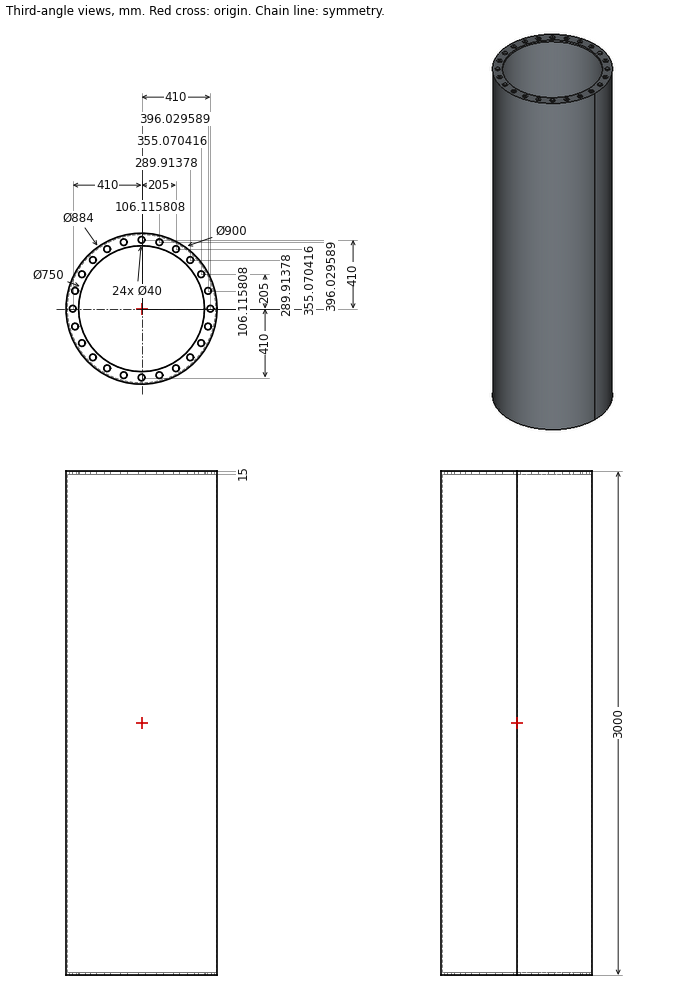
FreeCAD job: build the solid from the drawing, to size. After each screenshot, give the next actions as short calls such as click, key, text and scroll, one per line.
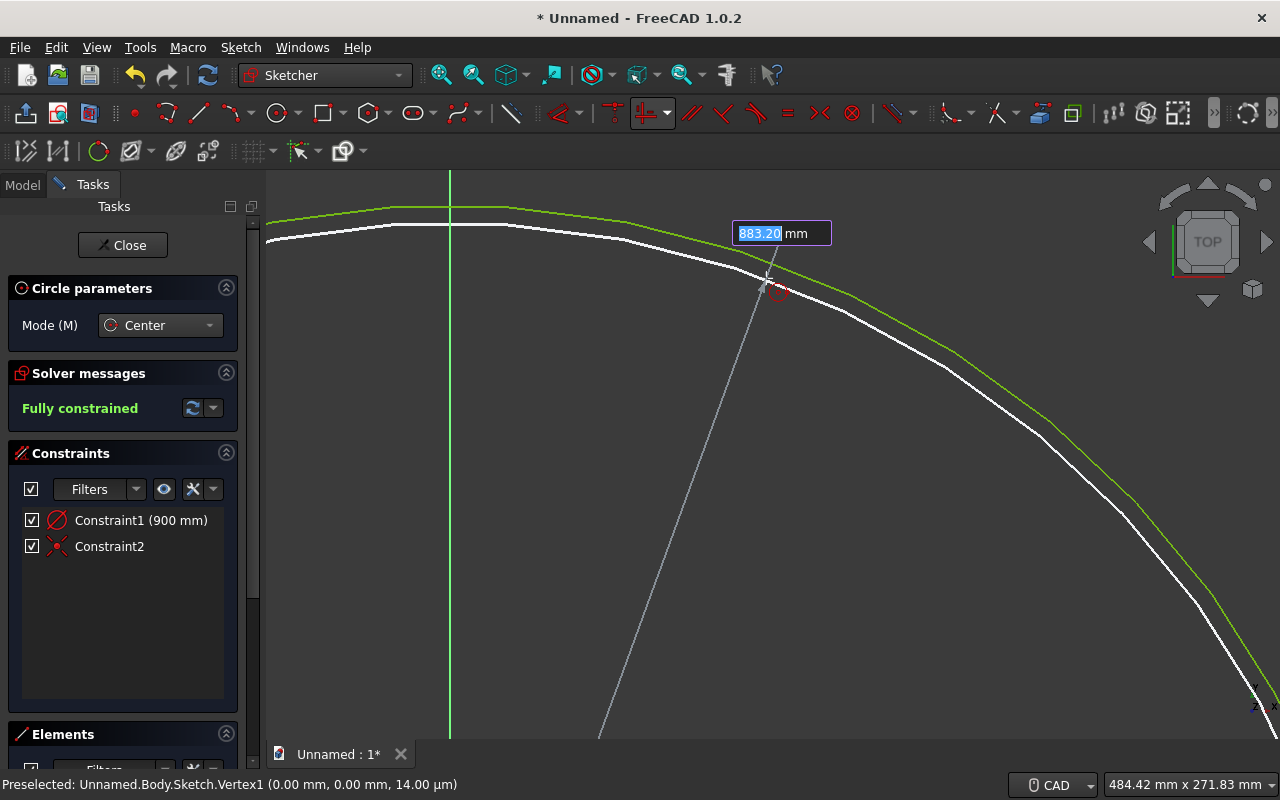
text(884)
key(Return)
key(Escape)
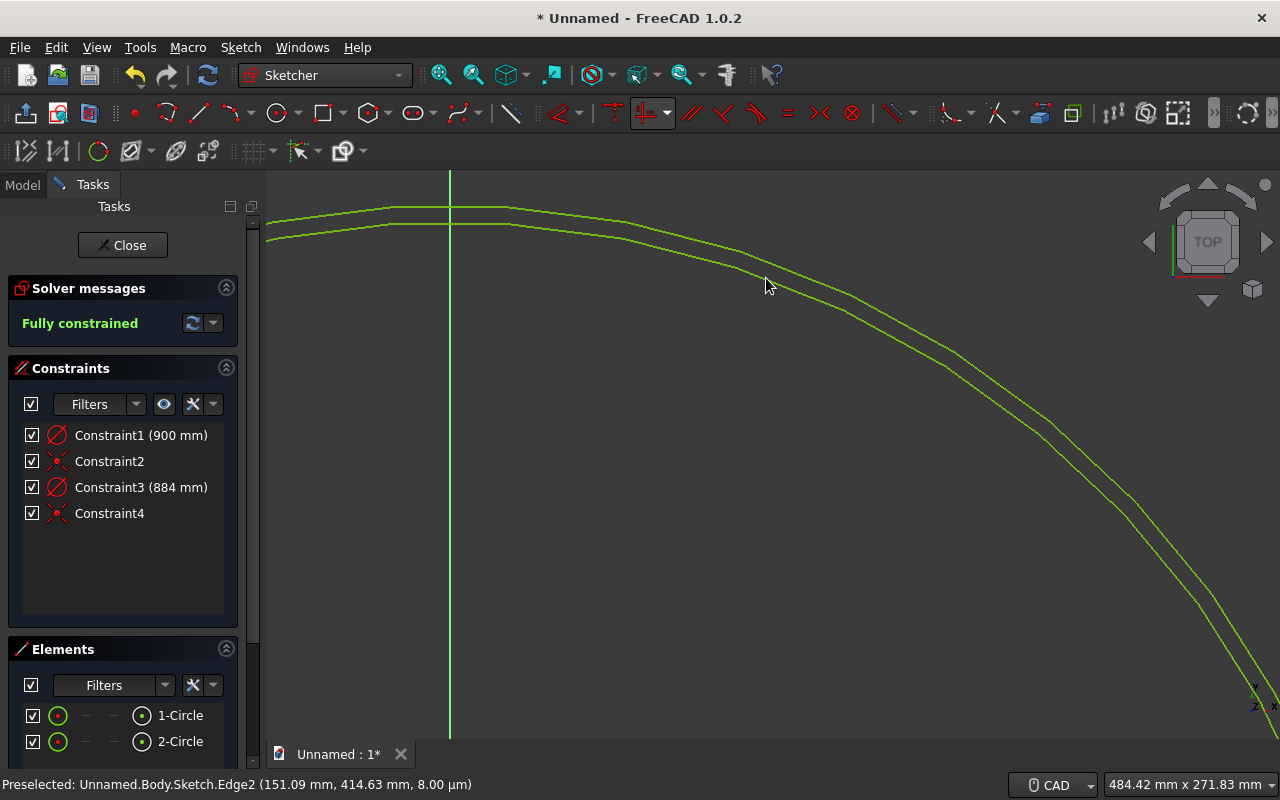
click(123, 245)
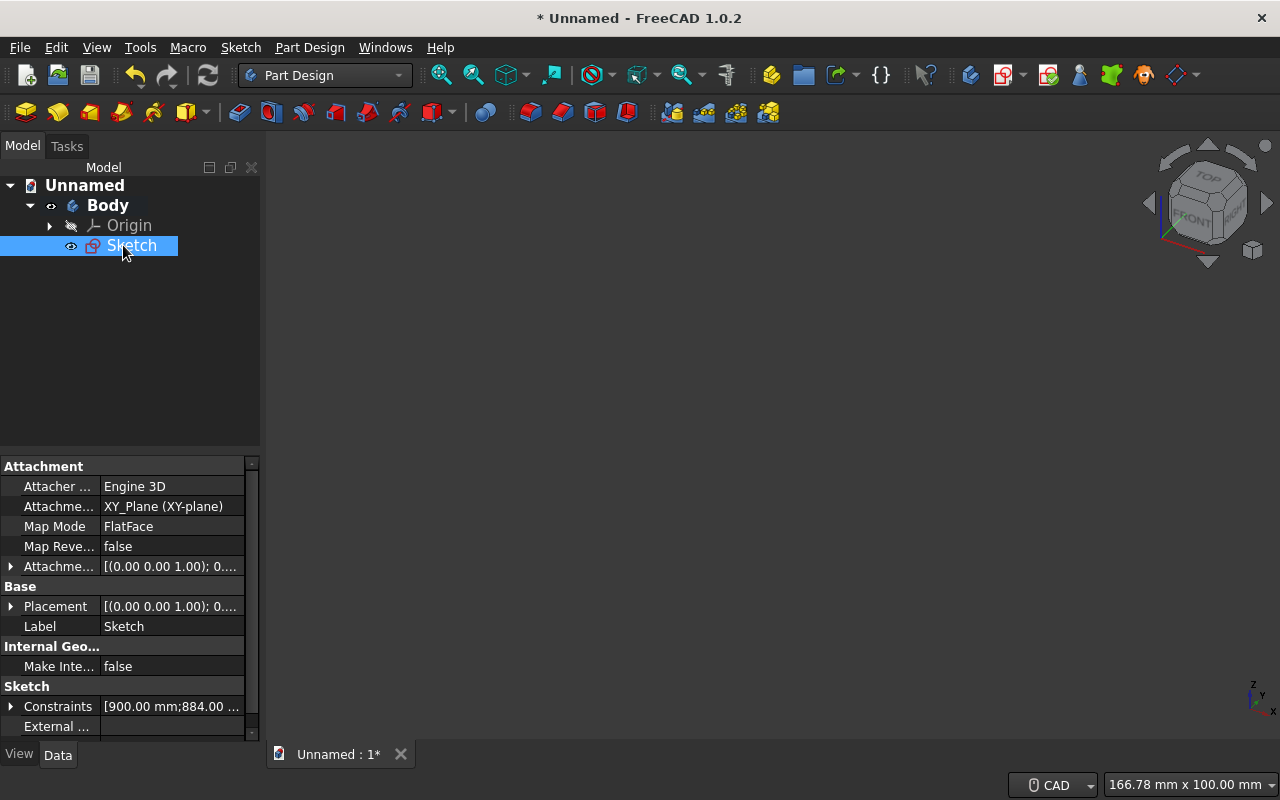
click(26, 112)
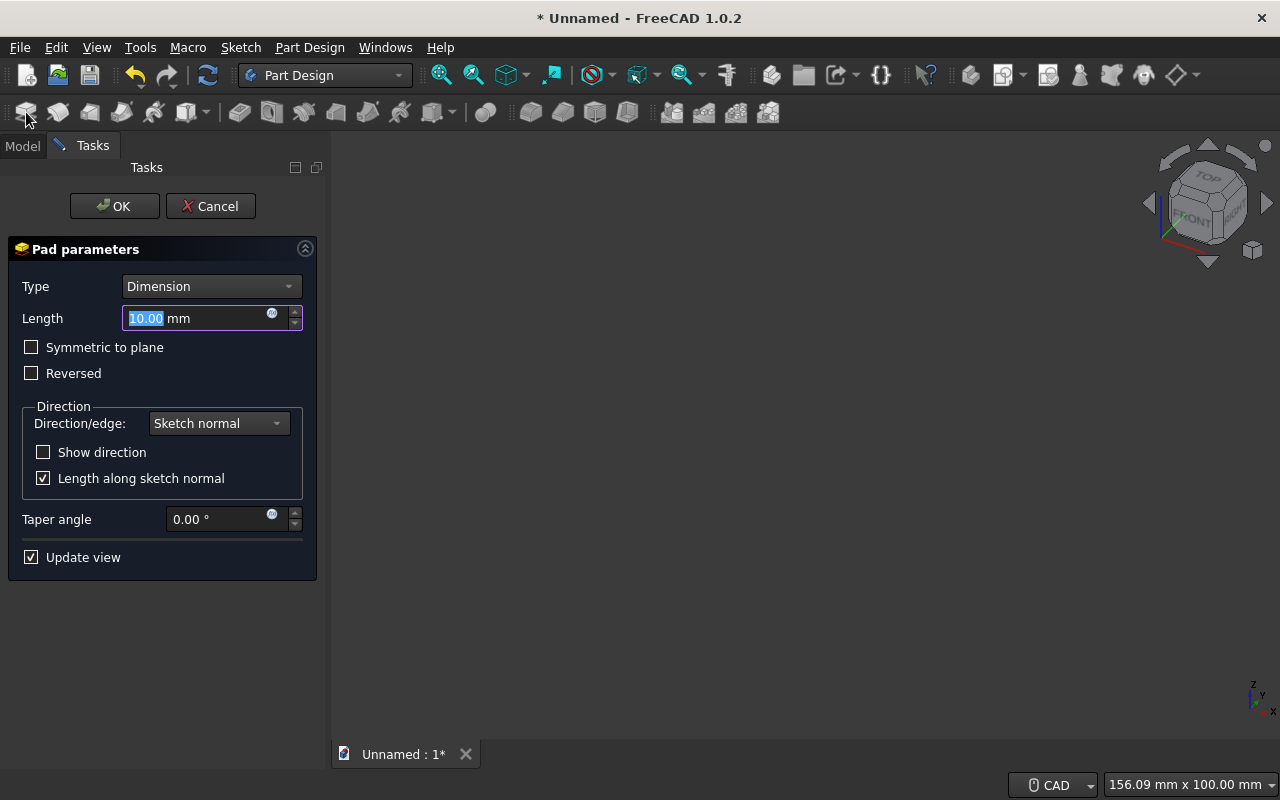
text(3000)
key(Tab)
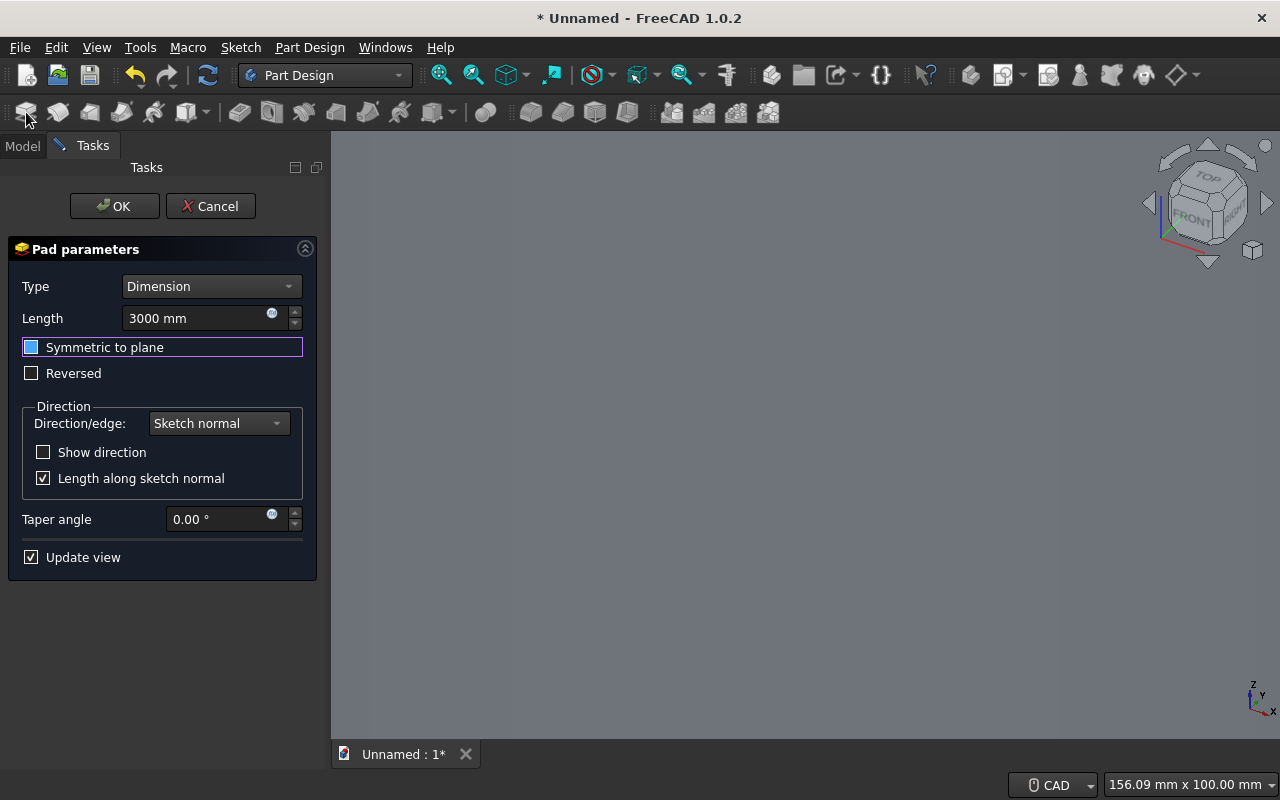
click(30, 347)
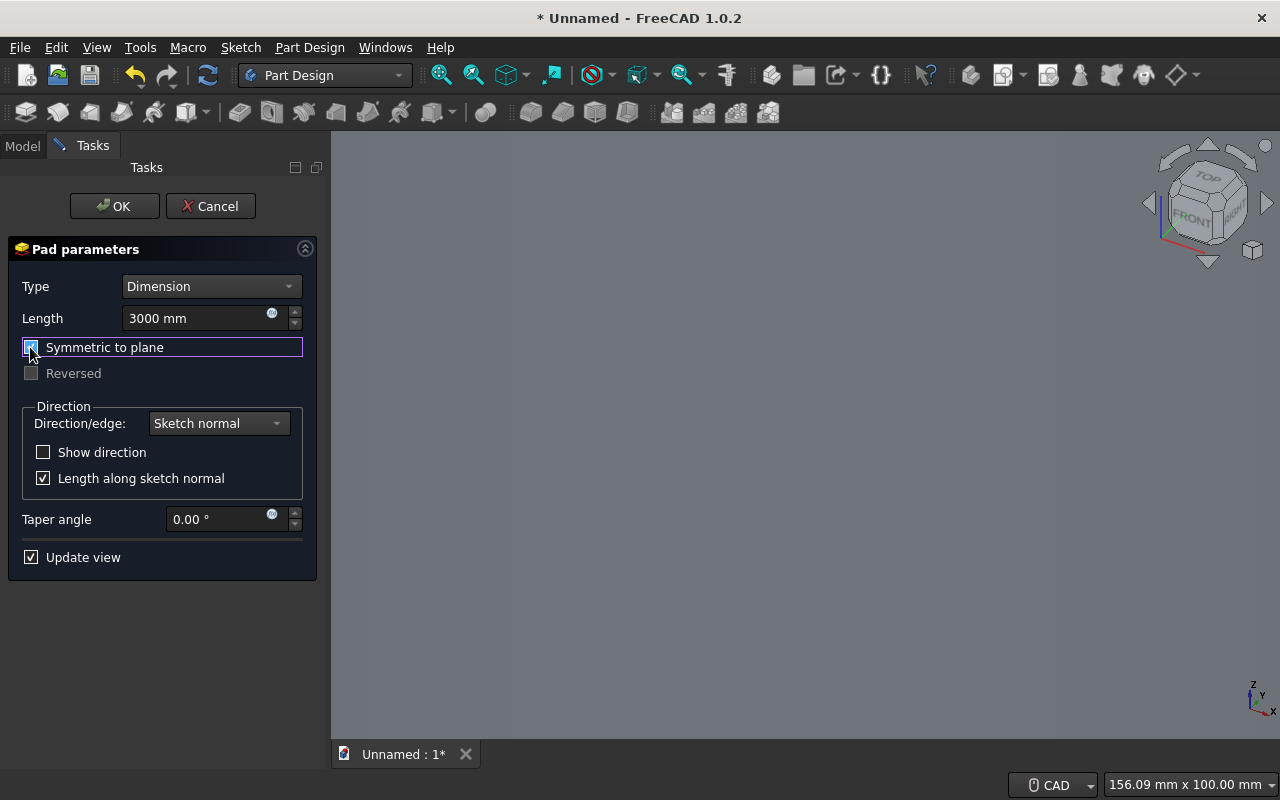
click(115, 206)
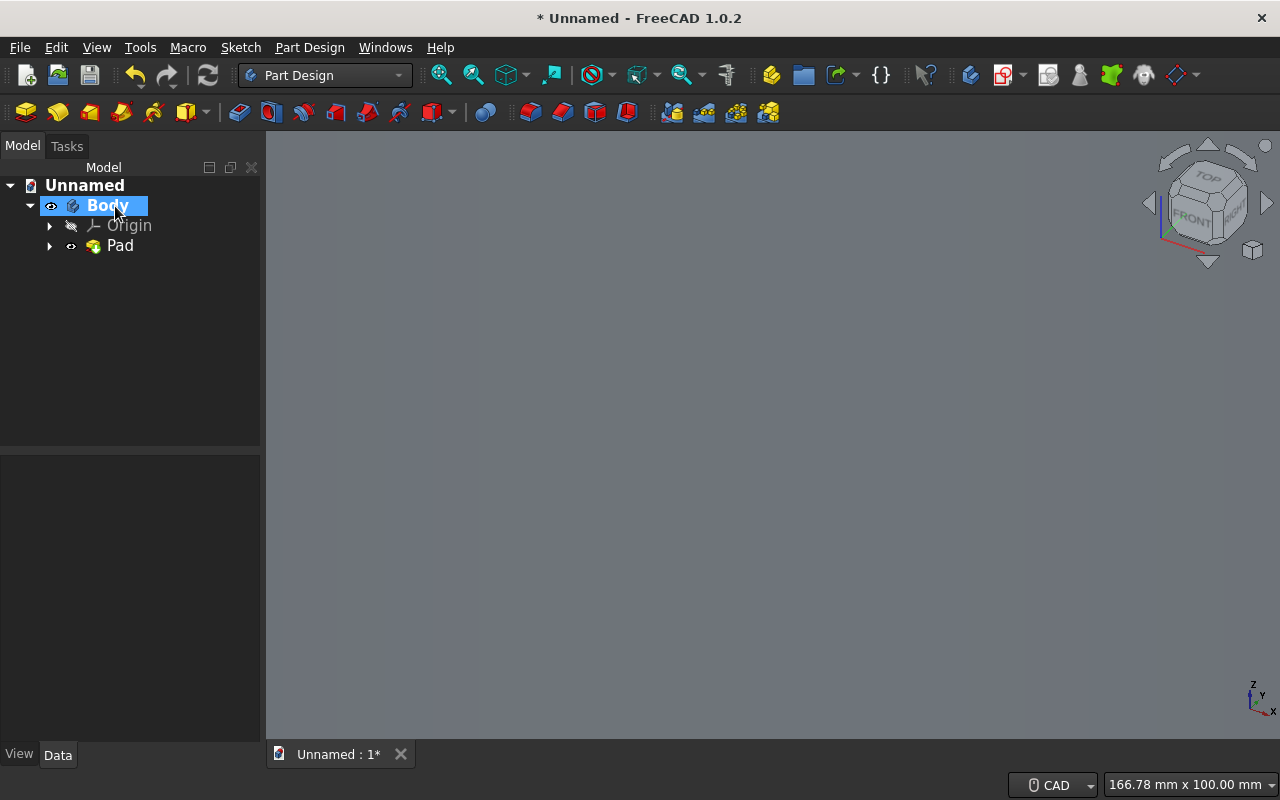
click(442, 76)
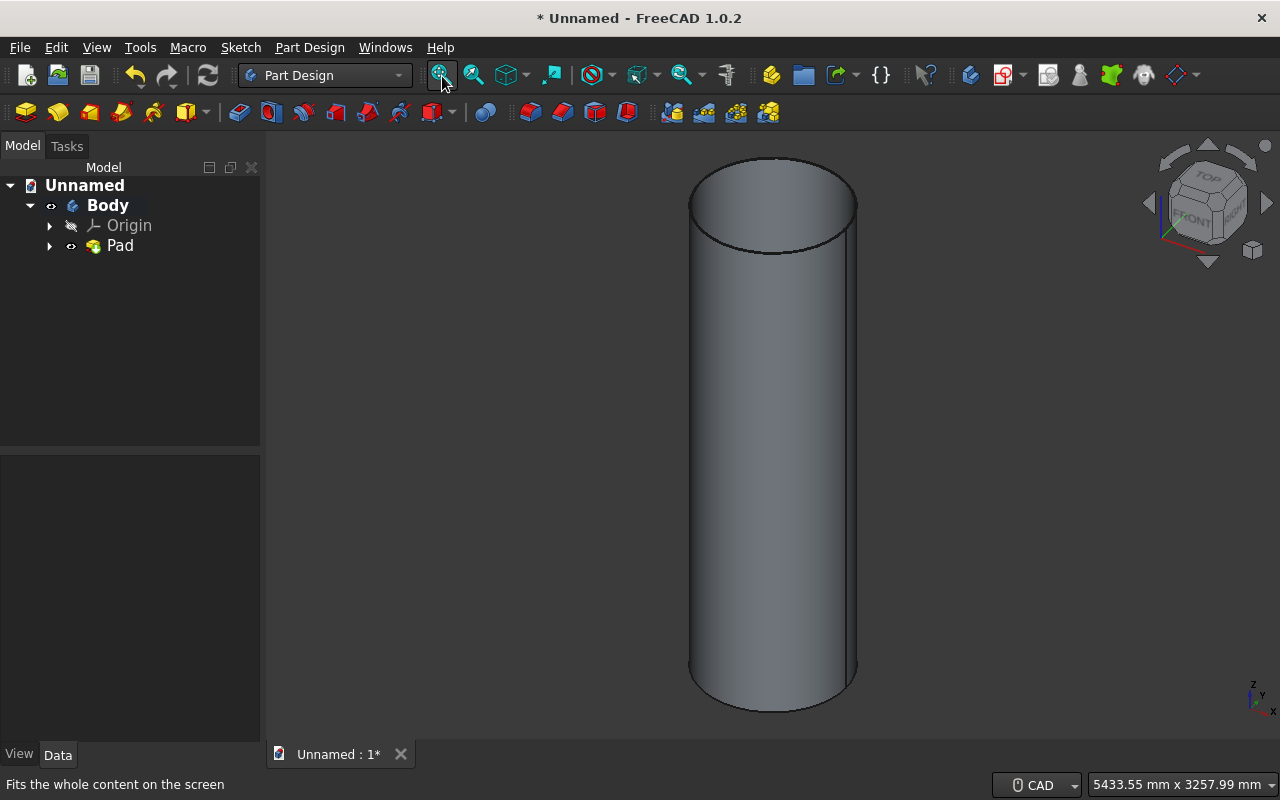
scroll(818, 164, up, 15)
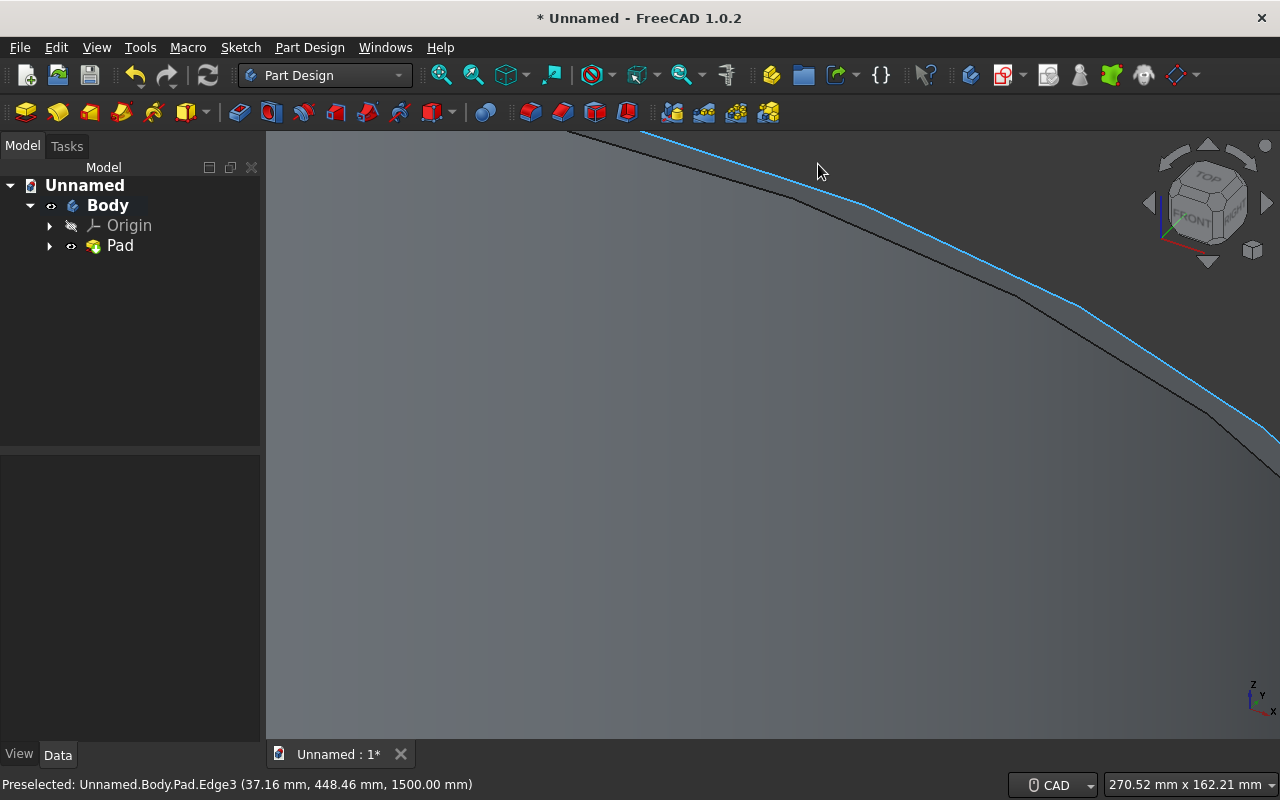
click(802, 188)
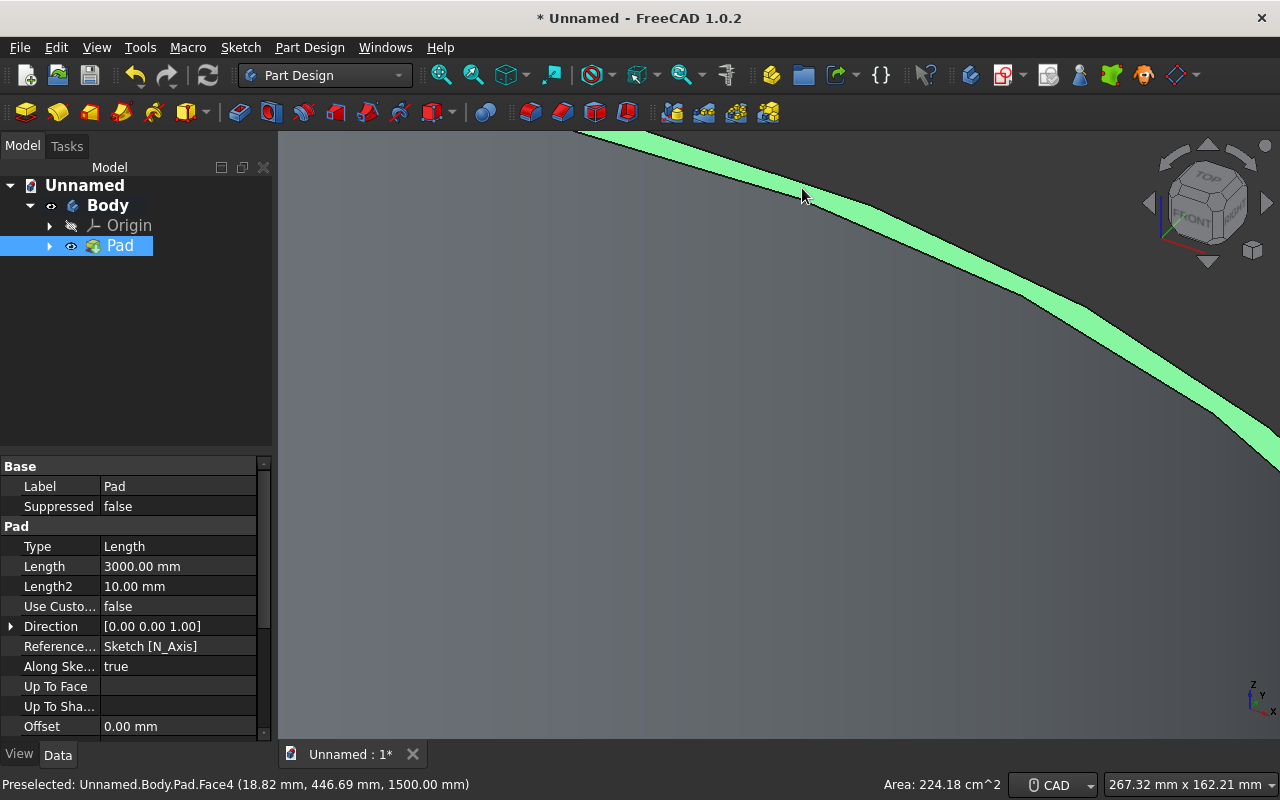
click(1004, 76)